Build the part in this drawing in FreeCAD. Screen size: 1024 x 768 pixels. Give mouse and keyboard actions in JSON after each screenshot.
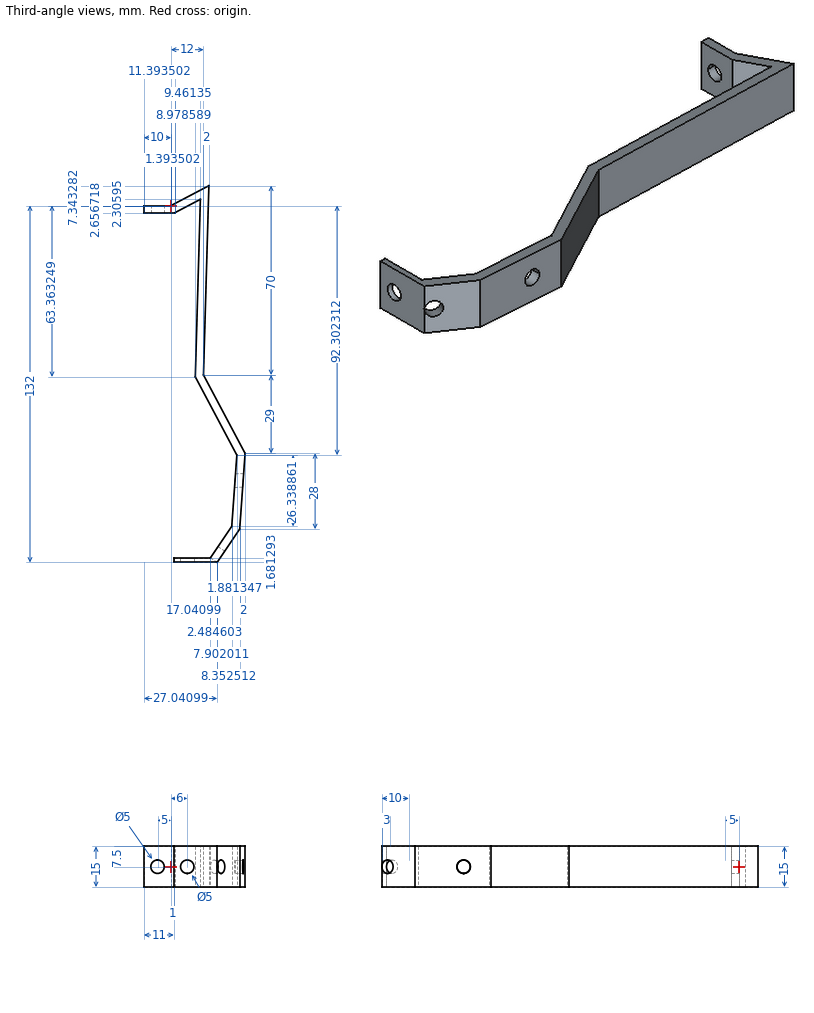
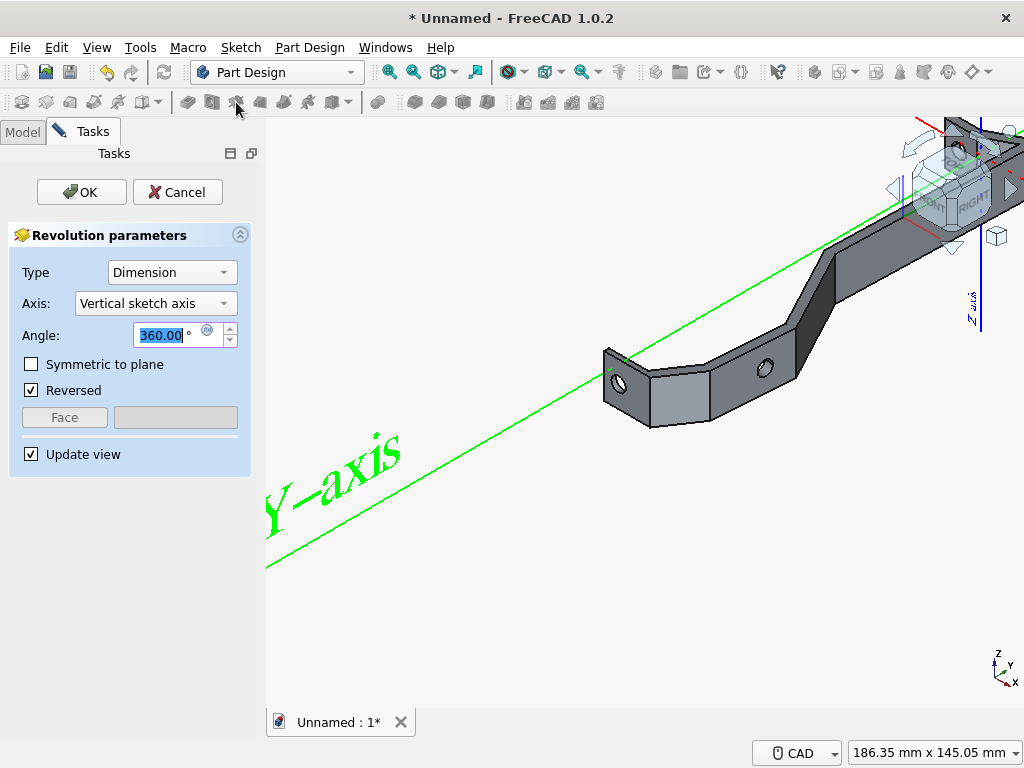
{"action": "left_click", "coordinate": [156, 304]}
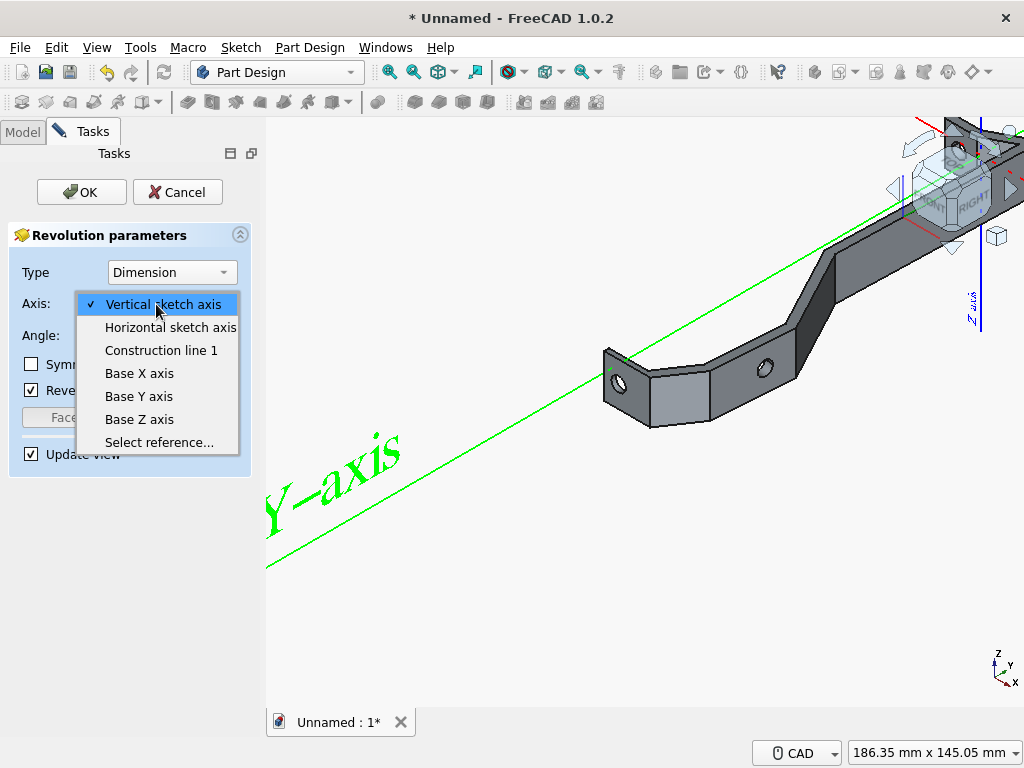
{"action": "left_click", "coordinate": [156, 350]}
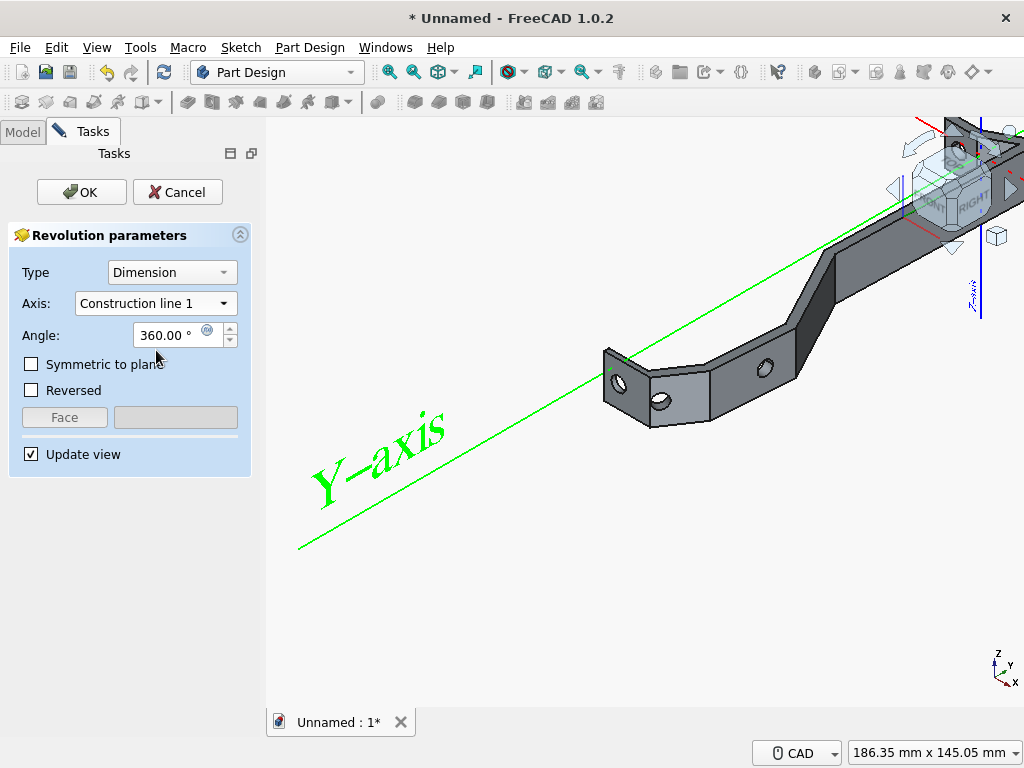
{"action": "left_click", "coordinate": [82, 192]}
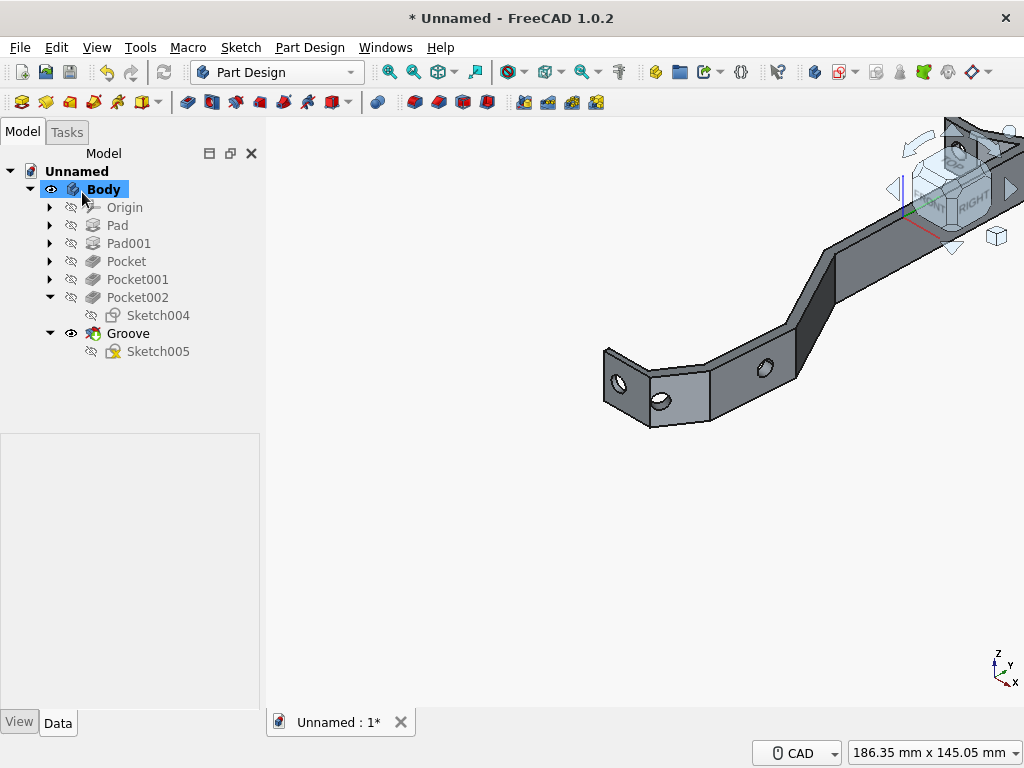
{"action": "left_click", "coordinate": [390, 72]}